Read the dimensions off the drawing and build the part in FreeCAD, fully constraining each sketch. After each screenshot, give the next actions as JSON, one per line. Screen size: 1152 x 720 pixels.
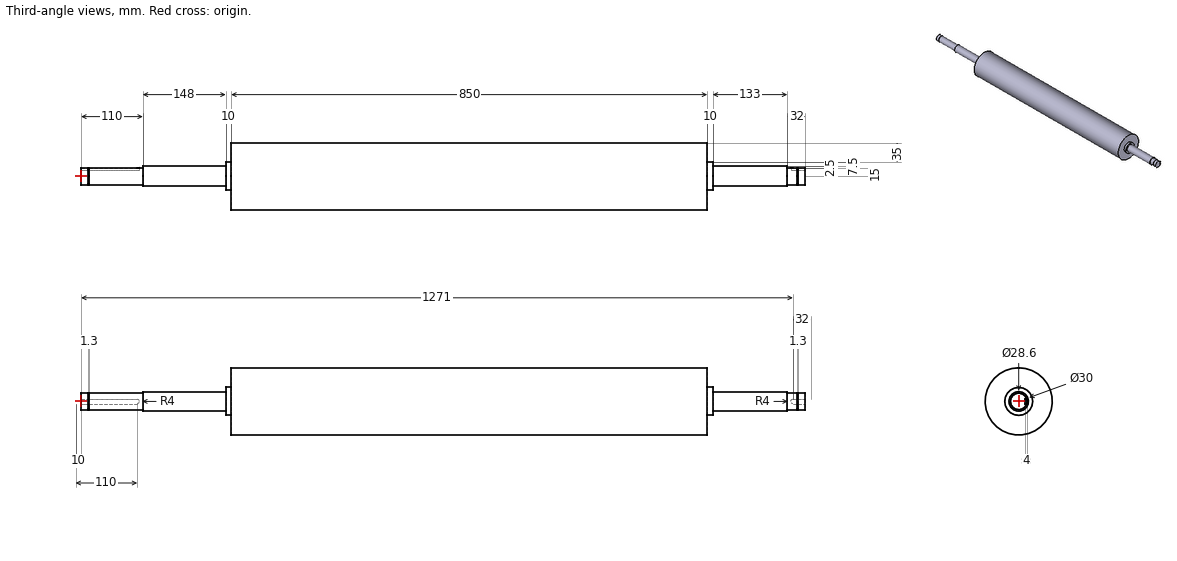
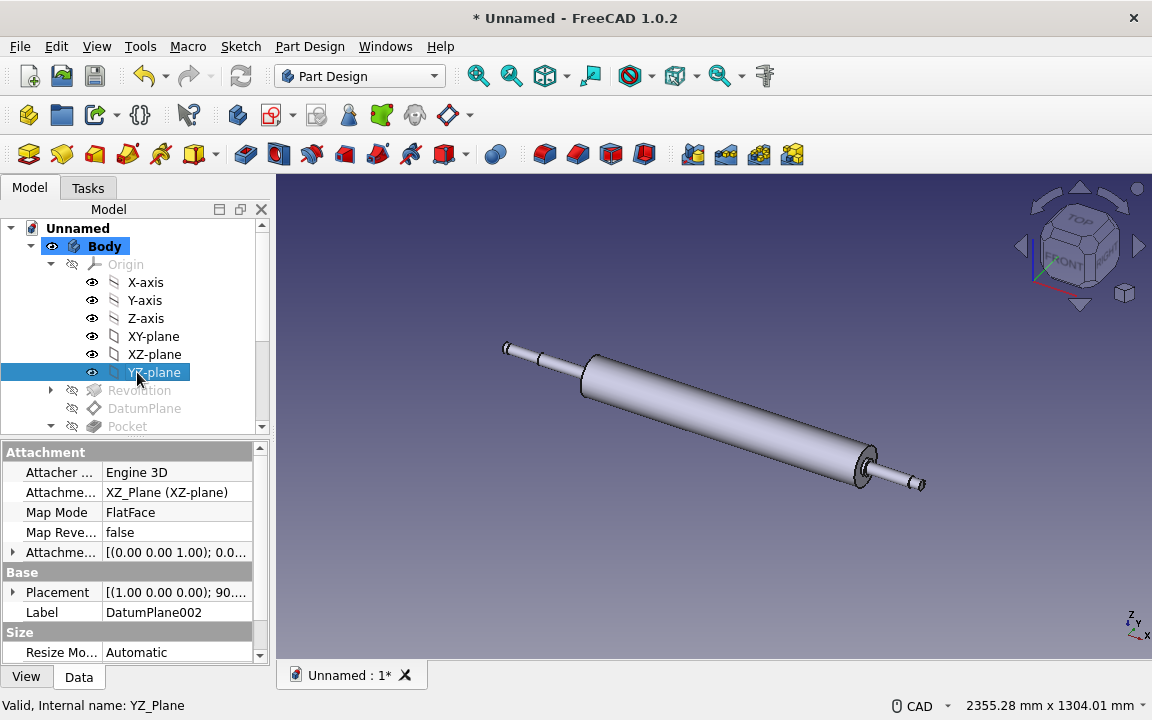
{"action": "left_click", "coordinate": [448, 116]}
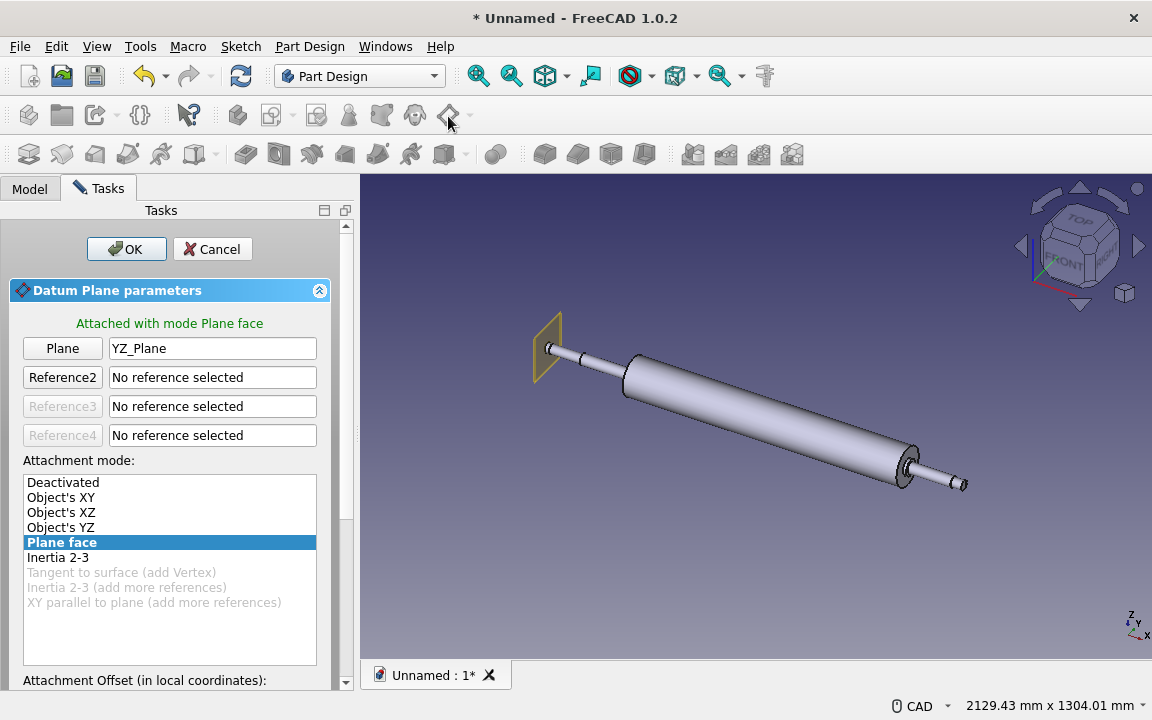
{"action": "scroll", "coordinate": [346, 455], "scroll_direction": "down", "scroll_amount": 3}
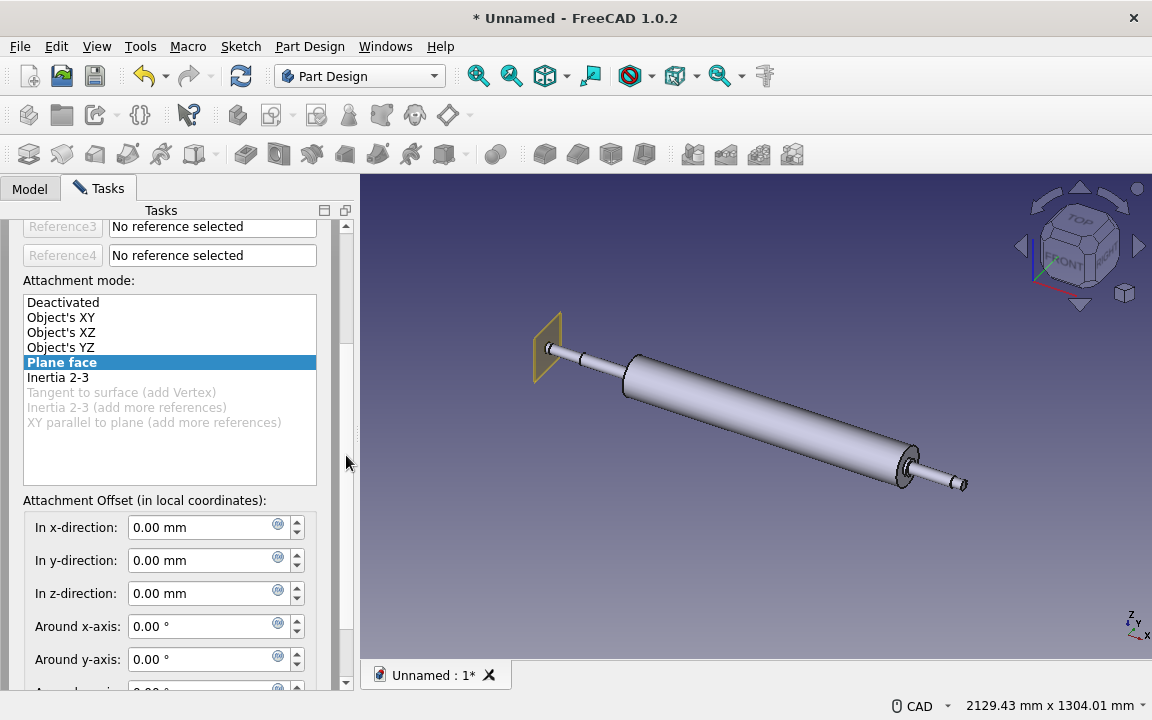
{"action": "triple_click", "coordinate": [210, 594]}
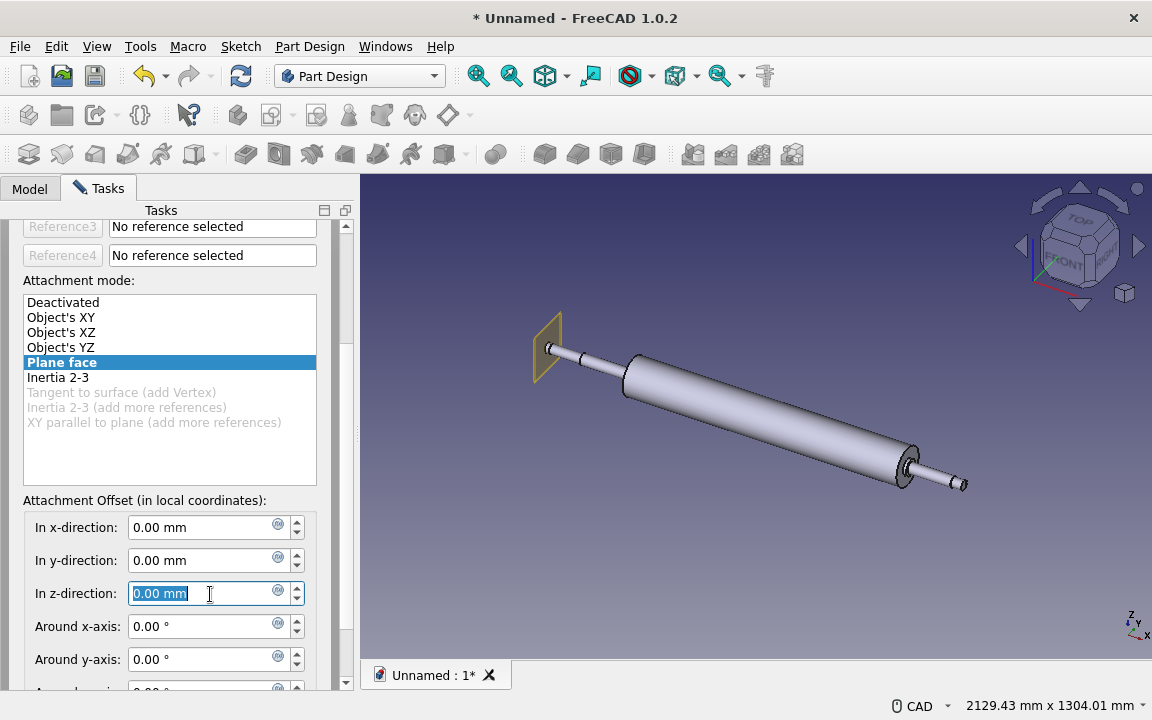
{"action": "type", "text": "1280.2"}
{"action": "key", "text": "Tab"}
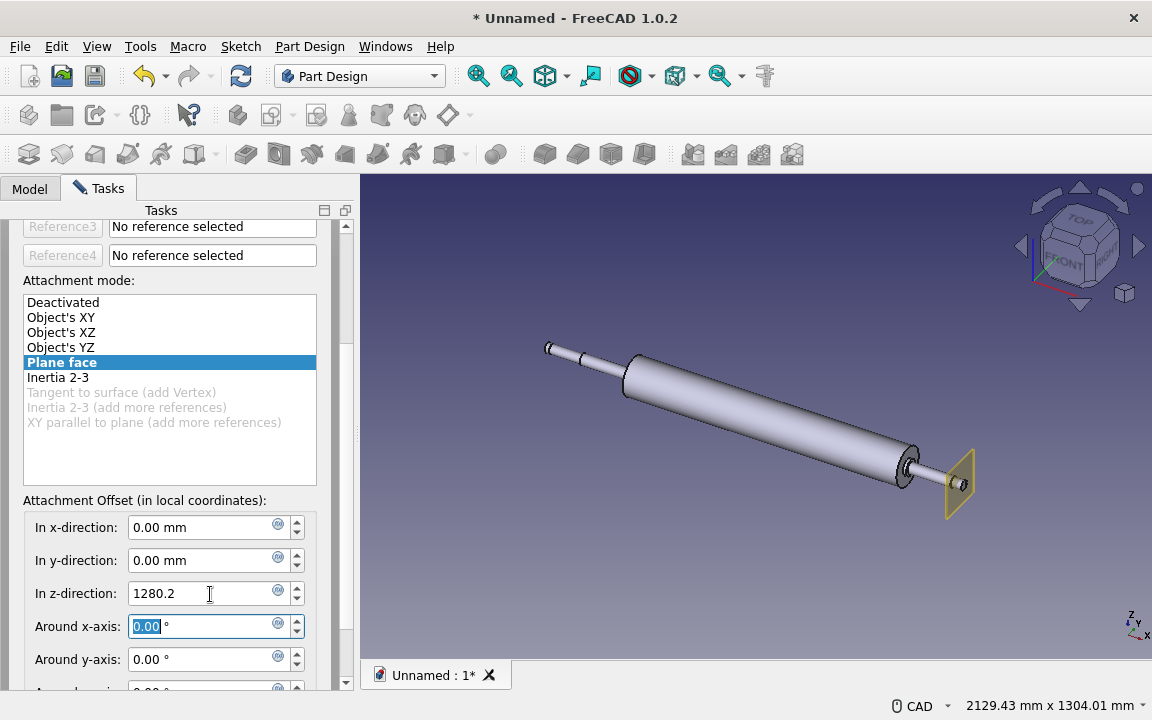
{"action": "scroll", "coordinate": [346, 455], "scroll_direction": "up", "scroll_amount": 4}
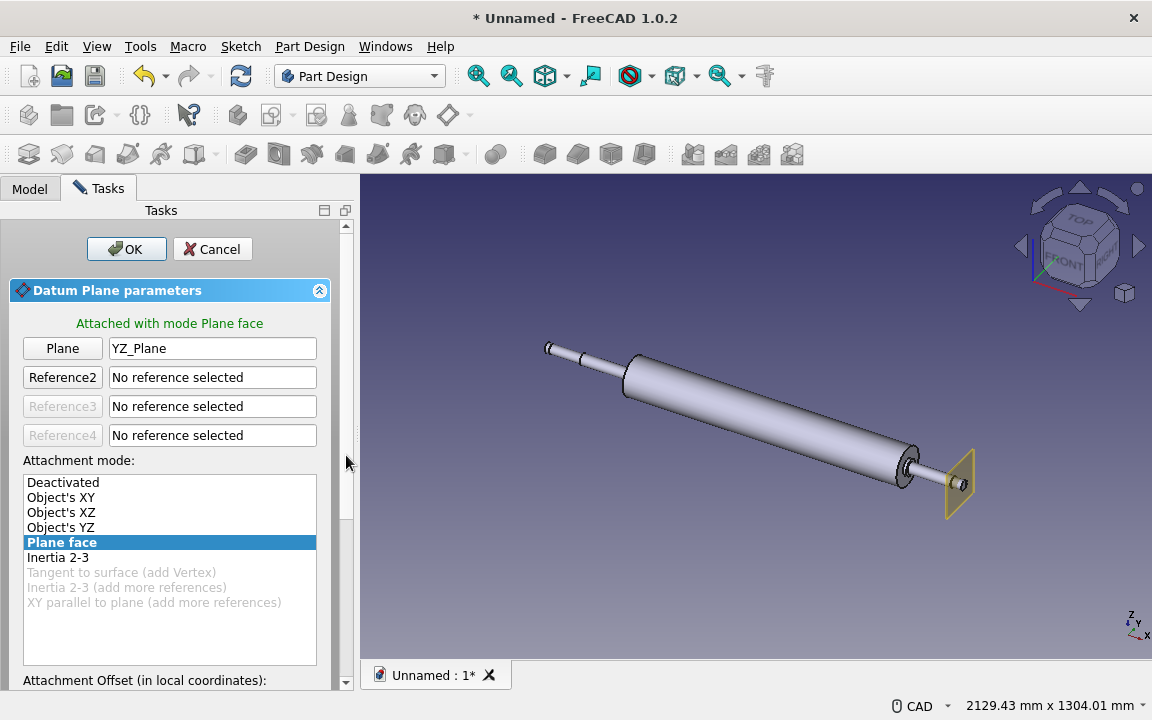
{"action": "left_click", "coordinate": [127, 249]}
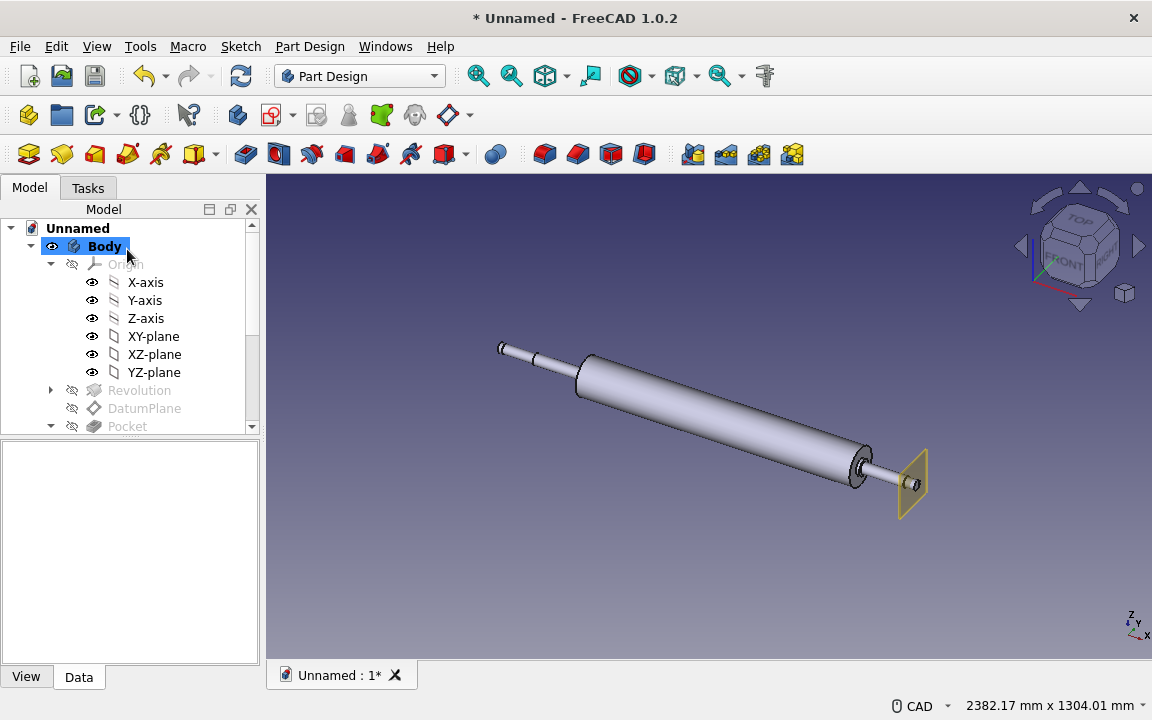
{"action": "scroll", "coordinate": [101, 332], "scroll_direction": "down", "scroll_amount": 3}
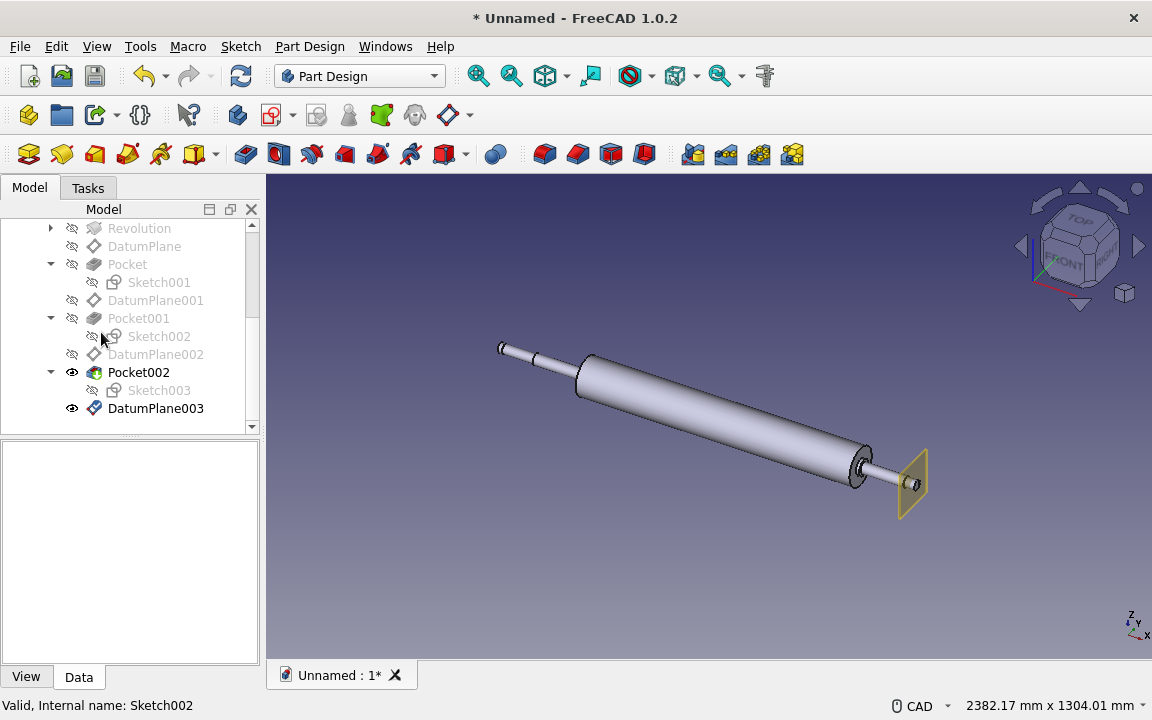
{"action": "left_click", "coordinate": [117, 408]}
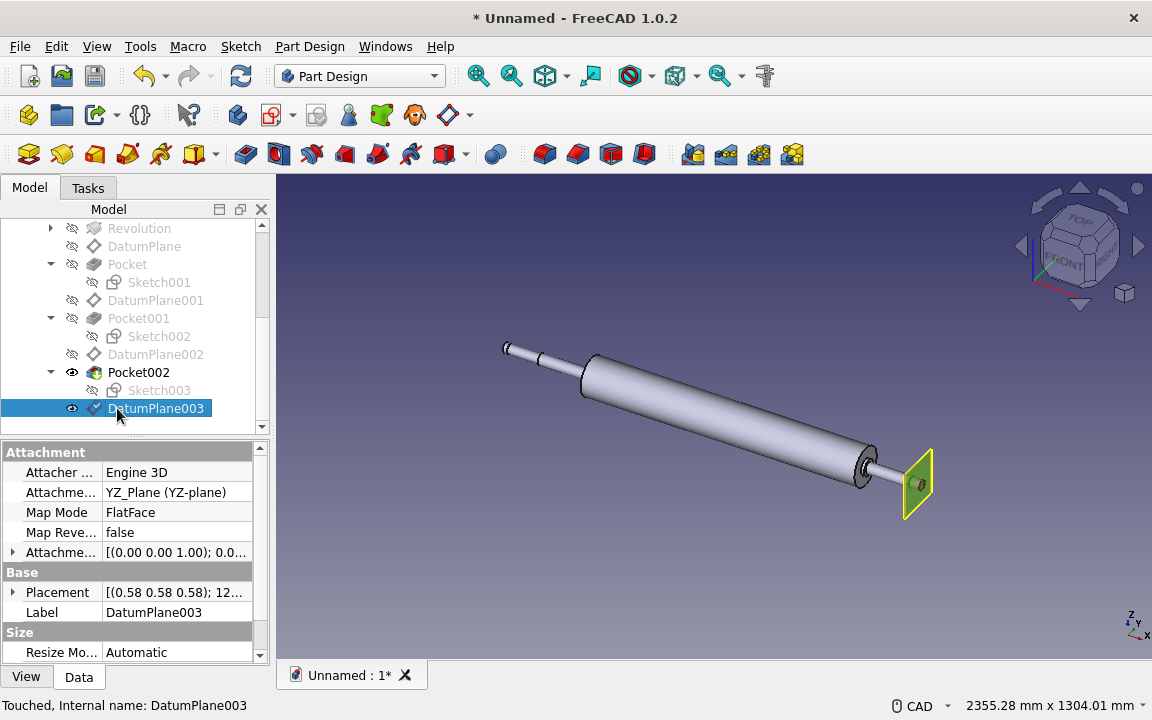
{"action": "left_click", "coordinate": [270, 116]}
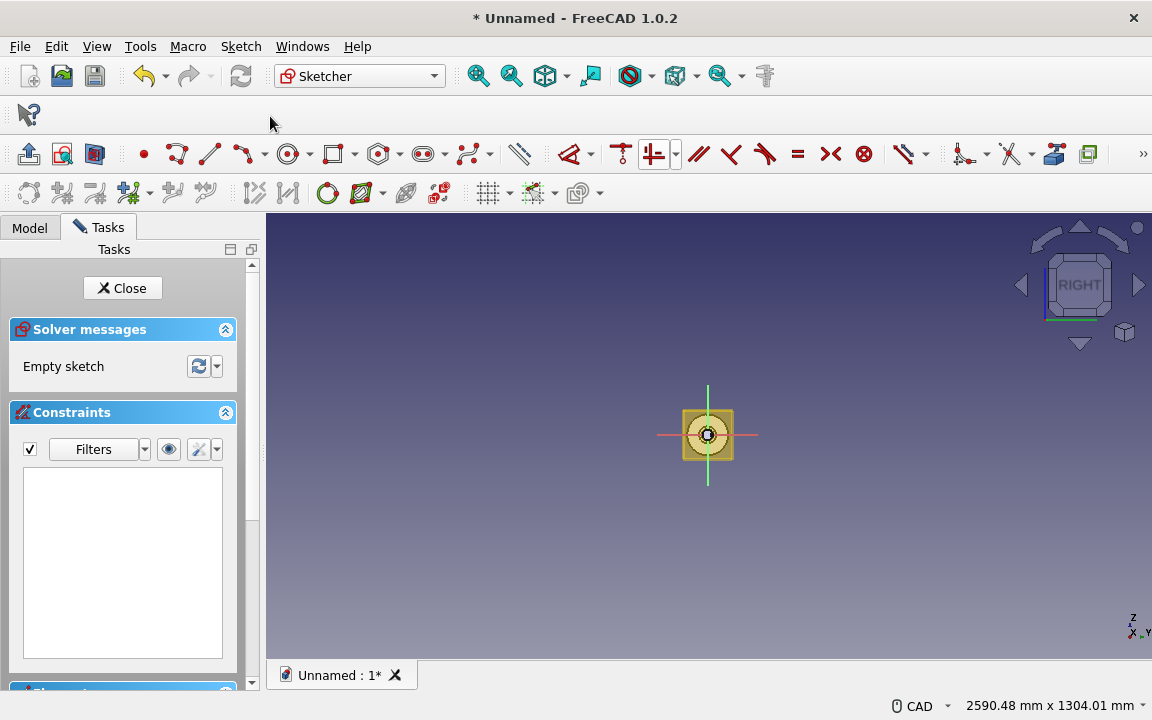
{"action": "left_click", "coordinate": [95, 154]}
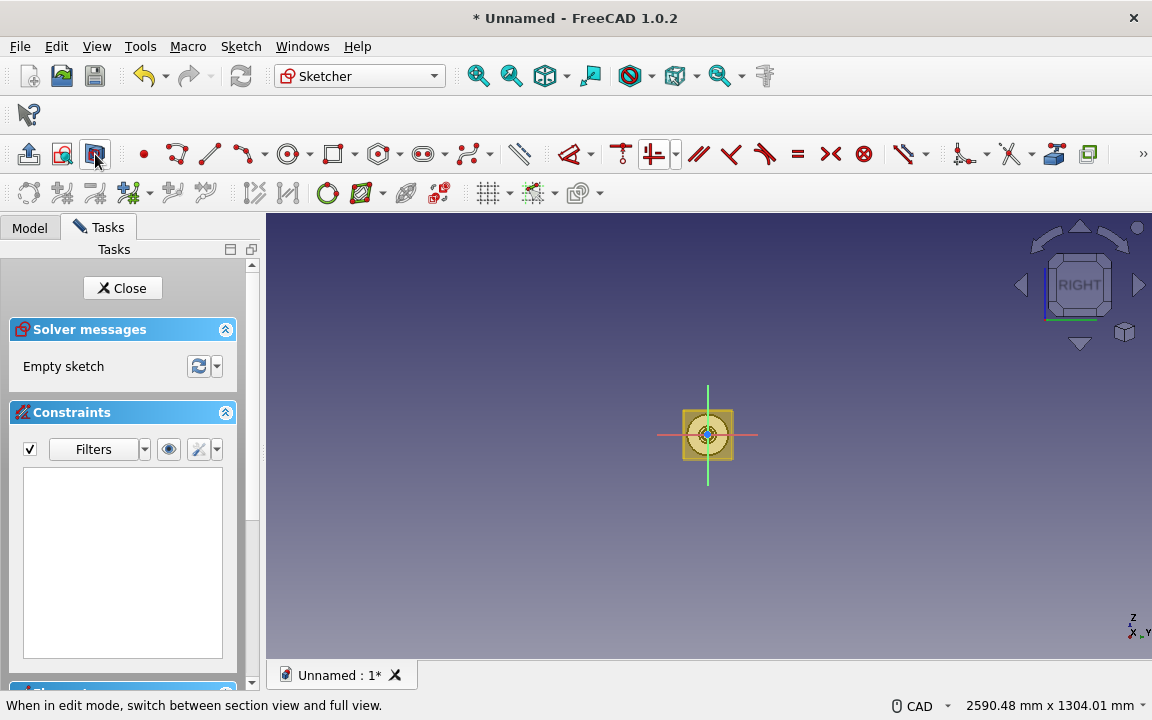
{"action": "scroll", "coordinate": [711, 435], "scroll_direction": "up", "scroll_amount": 15}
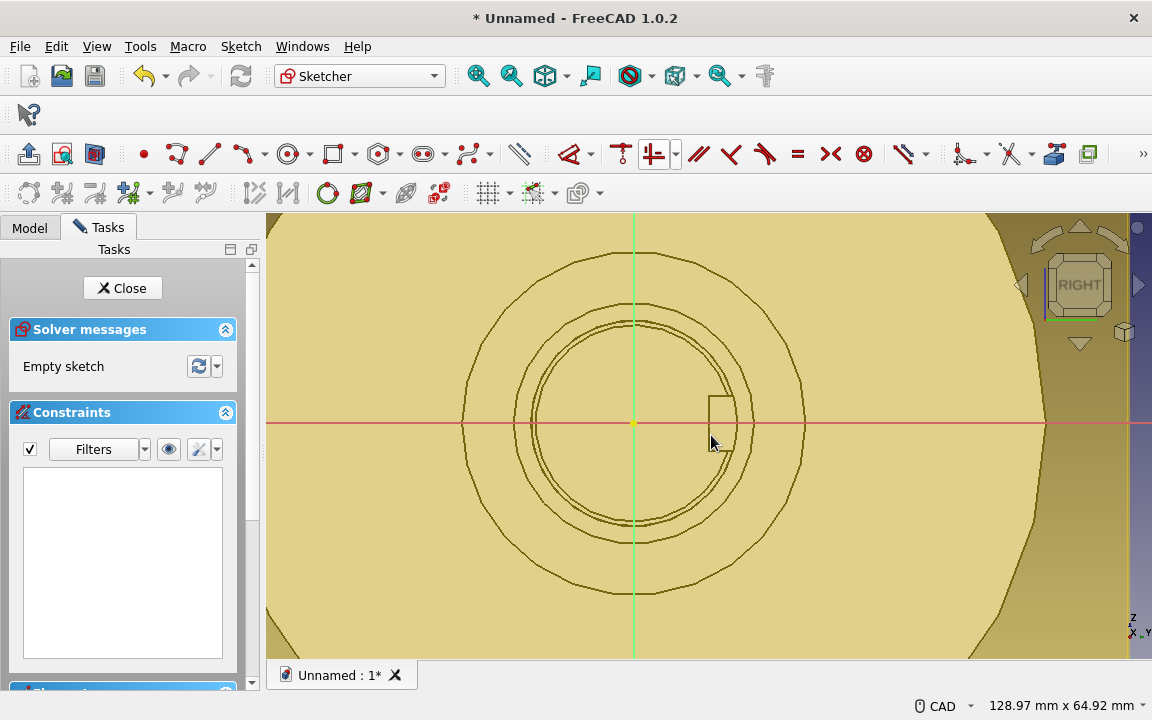
{"action": "key", "text": "g c"}